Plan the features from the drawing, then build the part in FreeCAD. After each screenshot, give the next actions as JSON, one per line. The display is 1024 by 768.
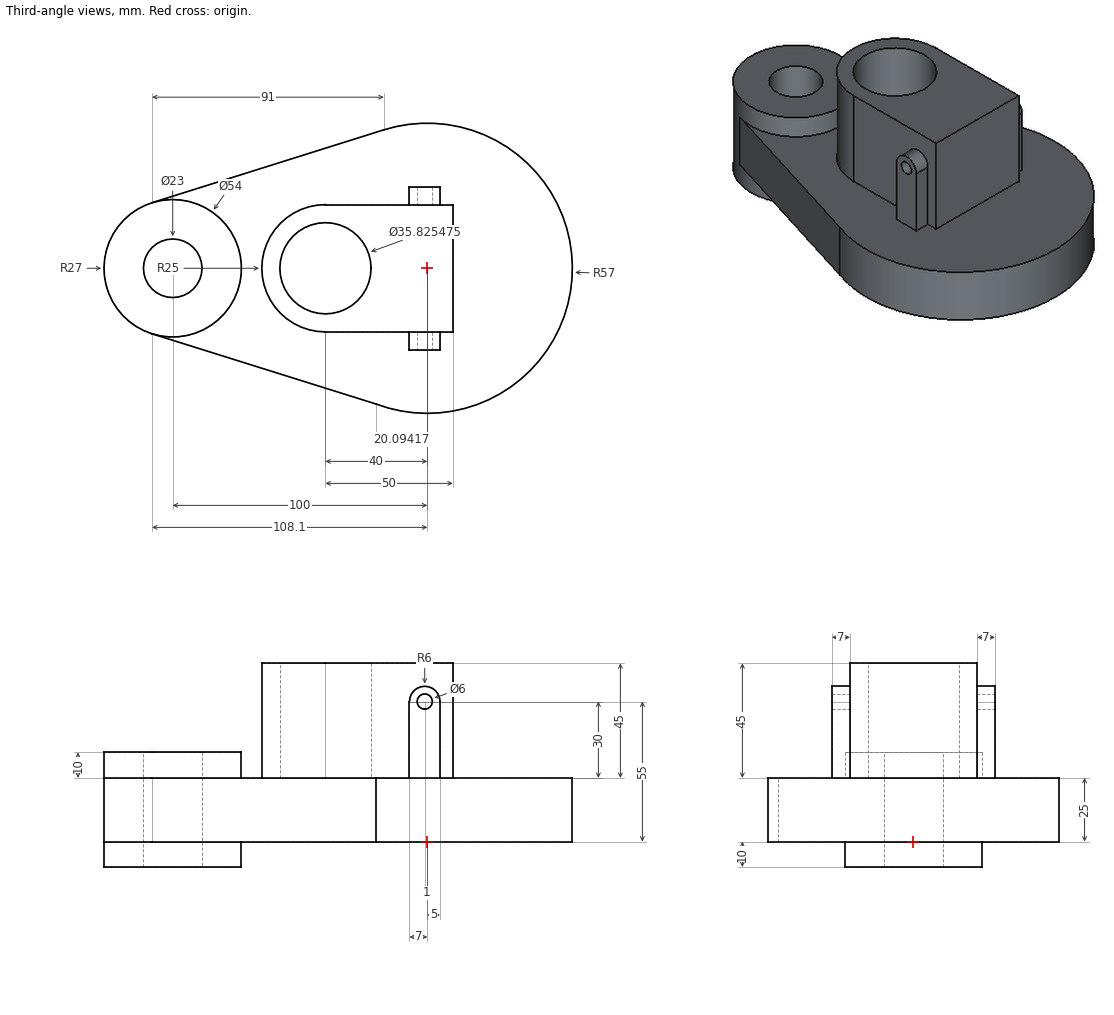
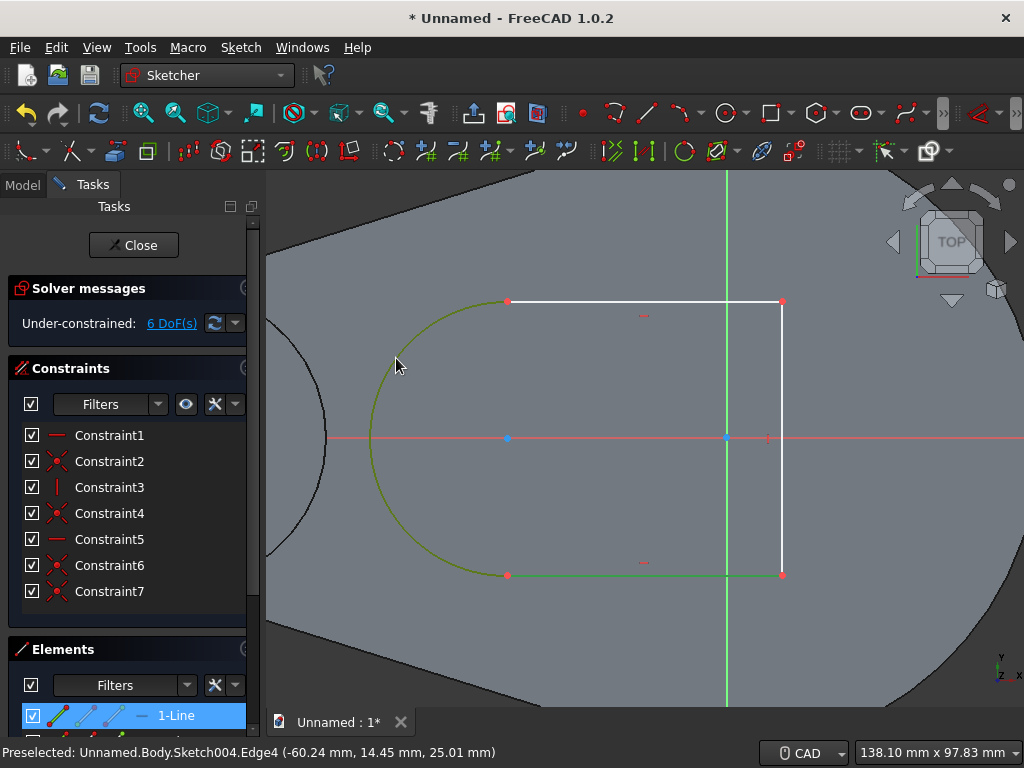
{"action": "key", "text": "t"}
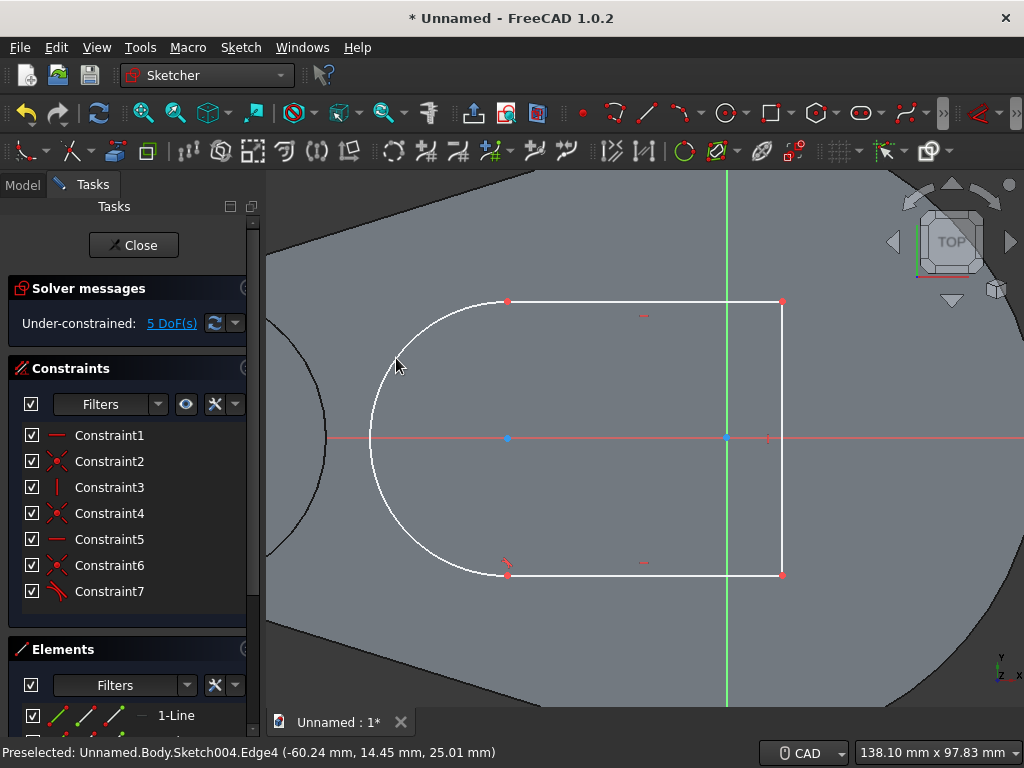
{"action": "left_click", "coordinate": [700, 302]}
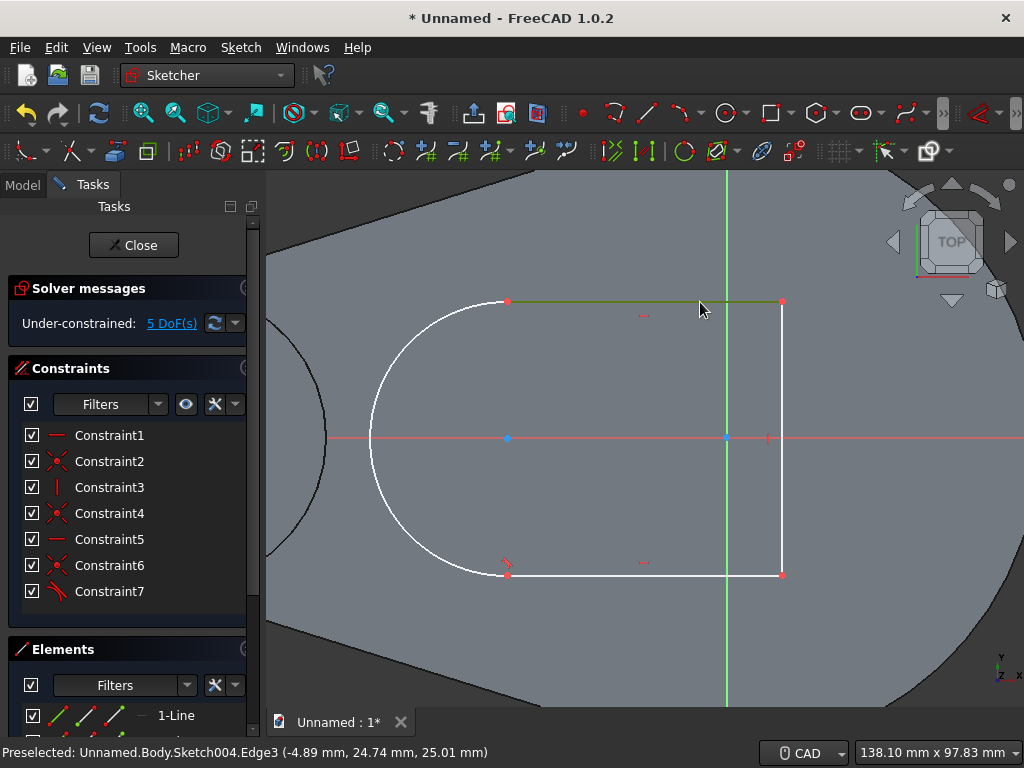
{"action": "left_click", "coordinate": [396, 359]}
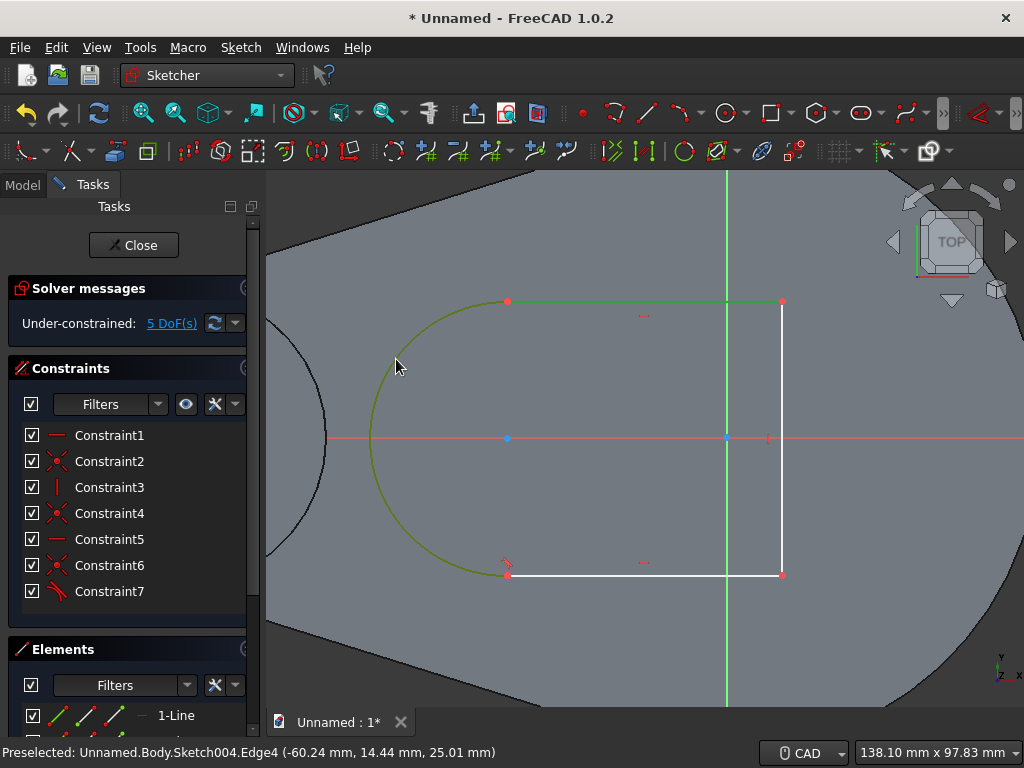
{"action": "key", "text": "t"}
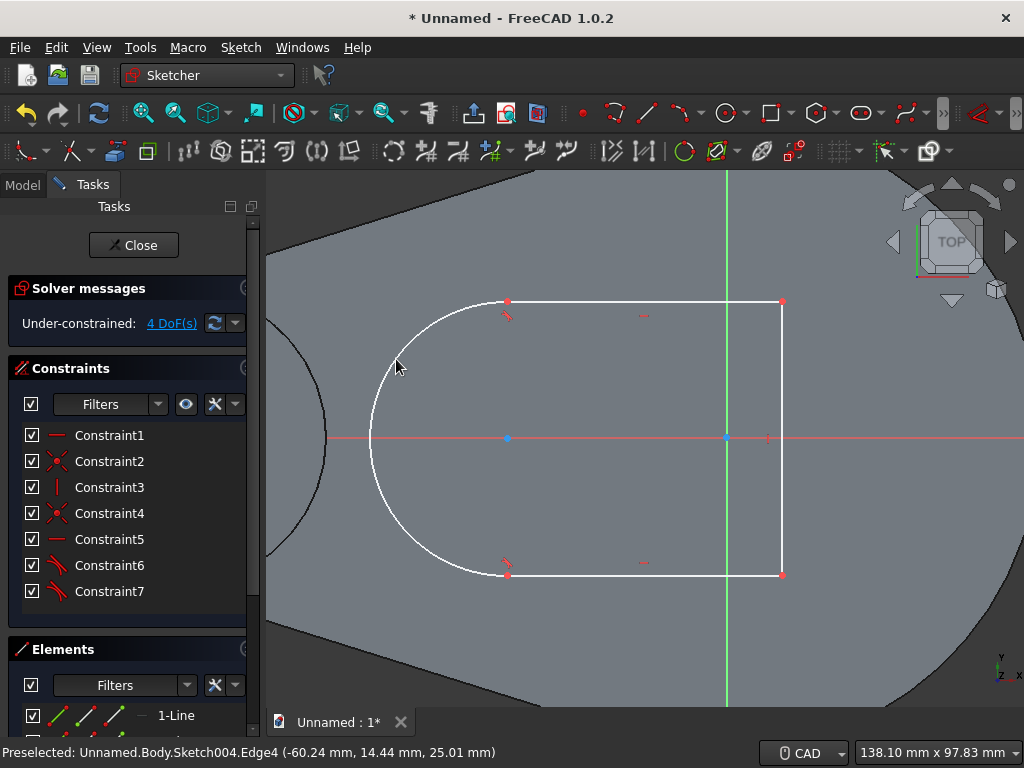
{"action": "left_click", "coordinate": [507, 439]}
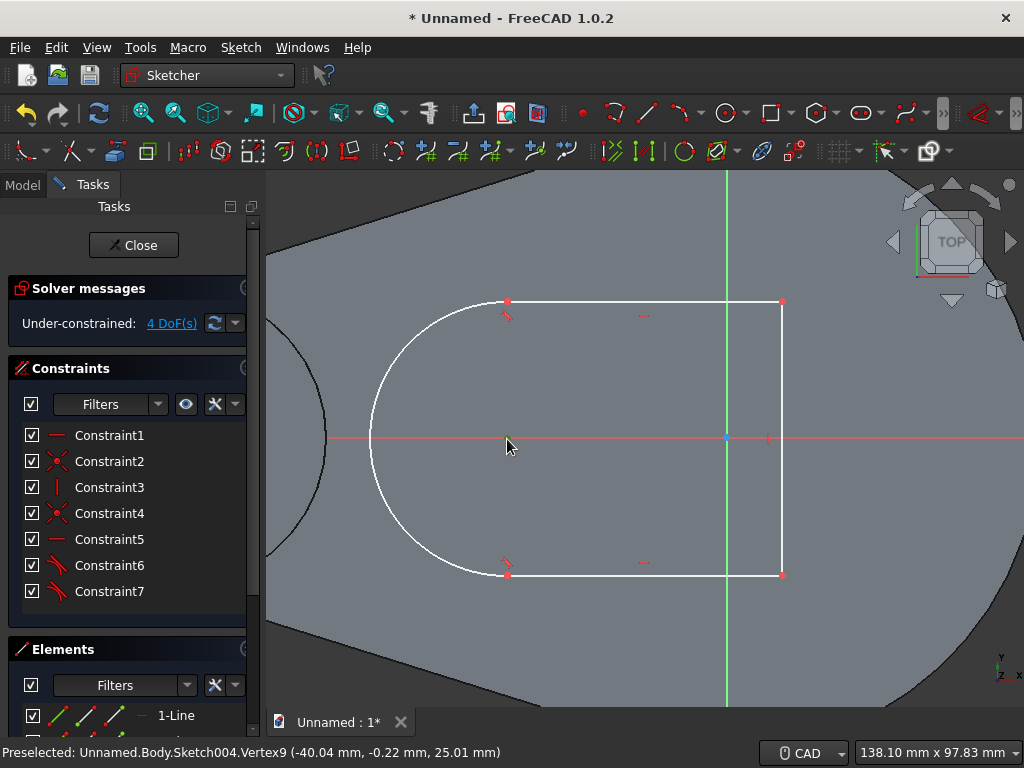
{"action": "left_click", "coordinate": [334, 438]}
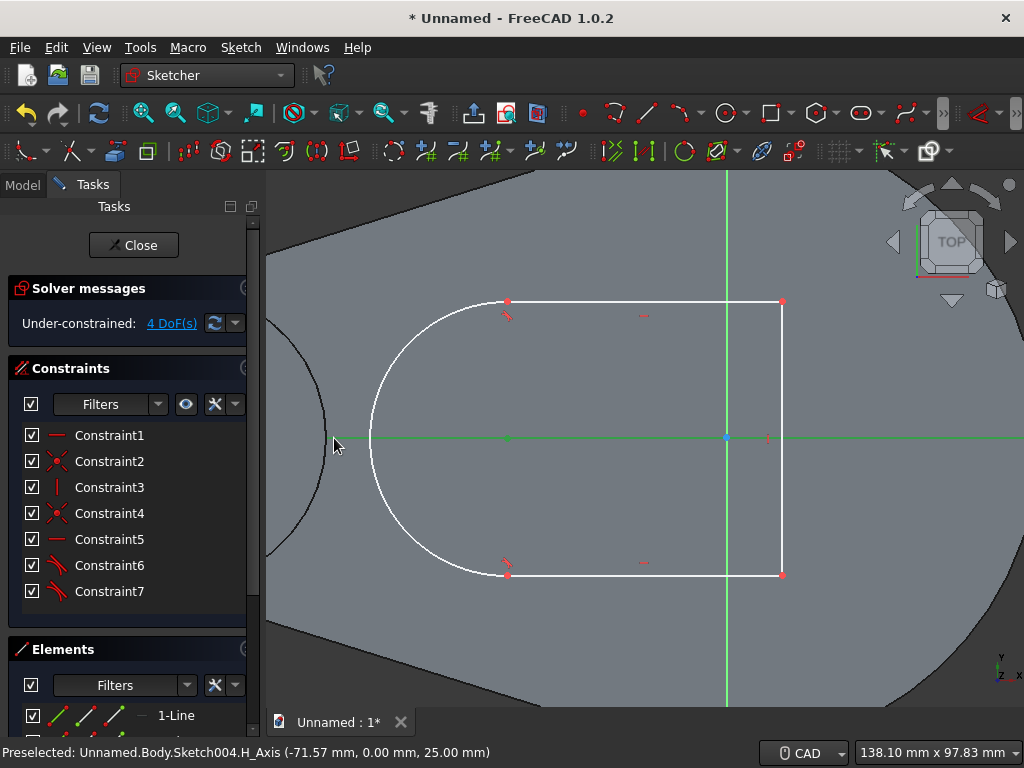
{"action": "key", "text": "c"}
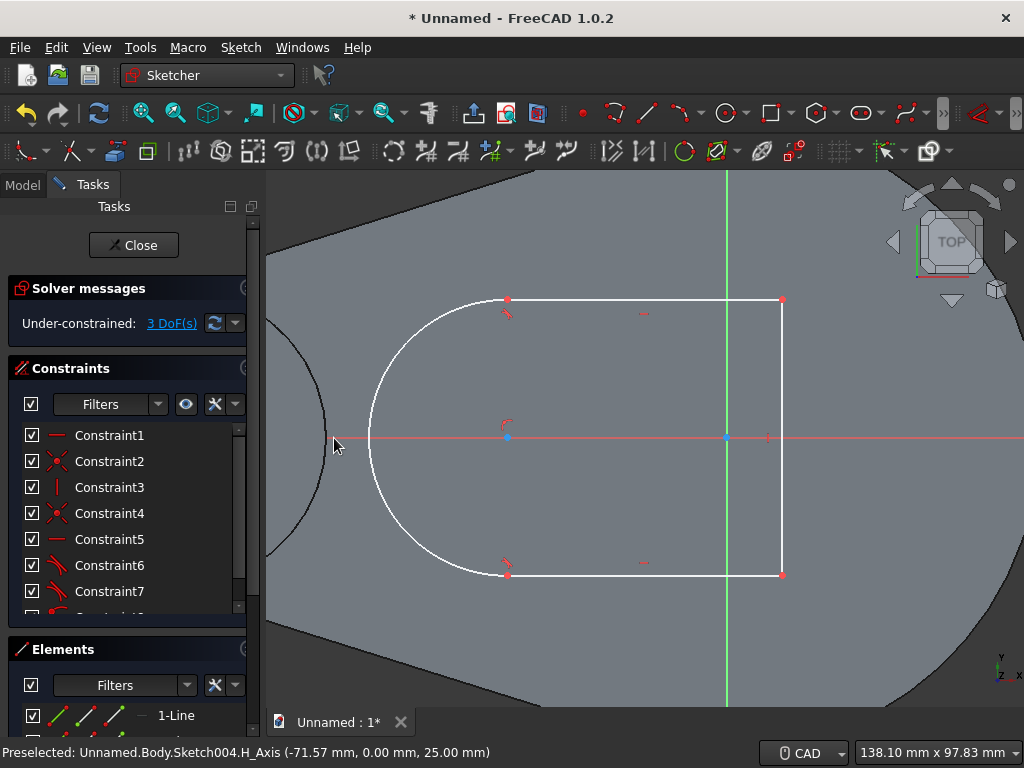
{"action": "left_click", "coordinate": [978, 114]}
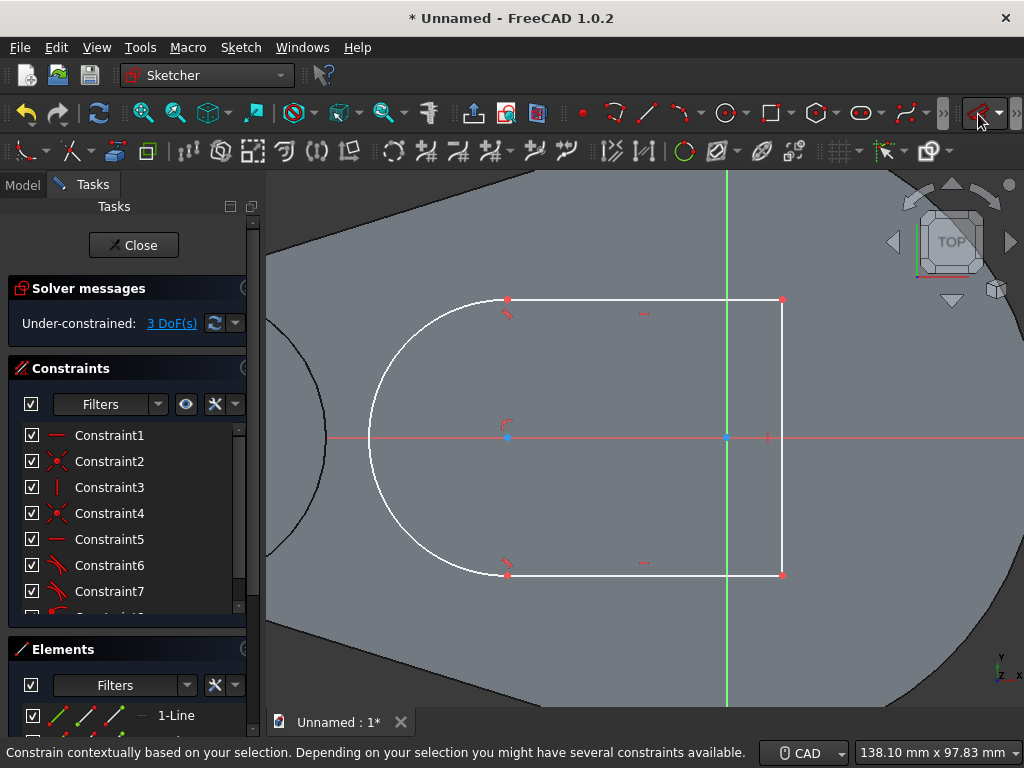
{"action": "left_click", "coordinate": [395, 357]}
{"action": "left_click", "coordinate": [369, 338]}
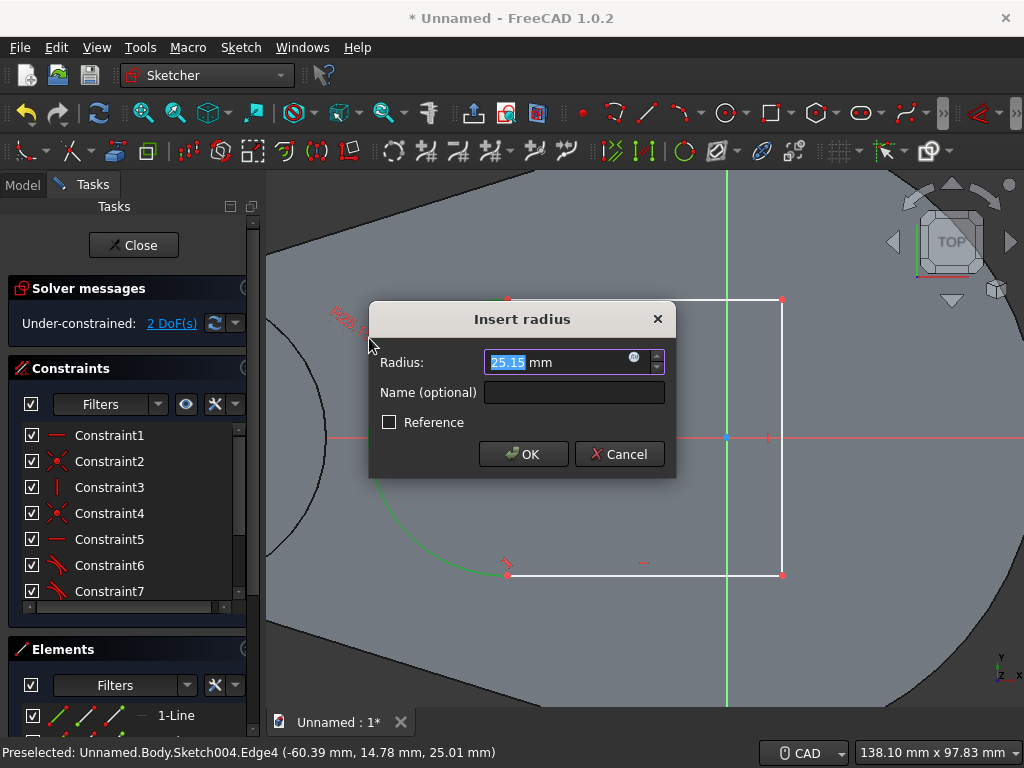
{"action": "type", "text": "25"}
{"action": "key", "text": "Return"}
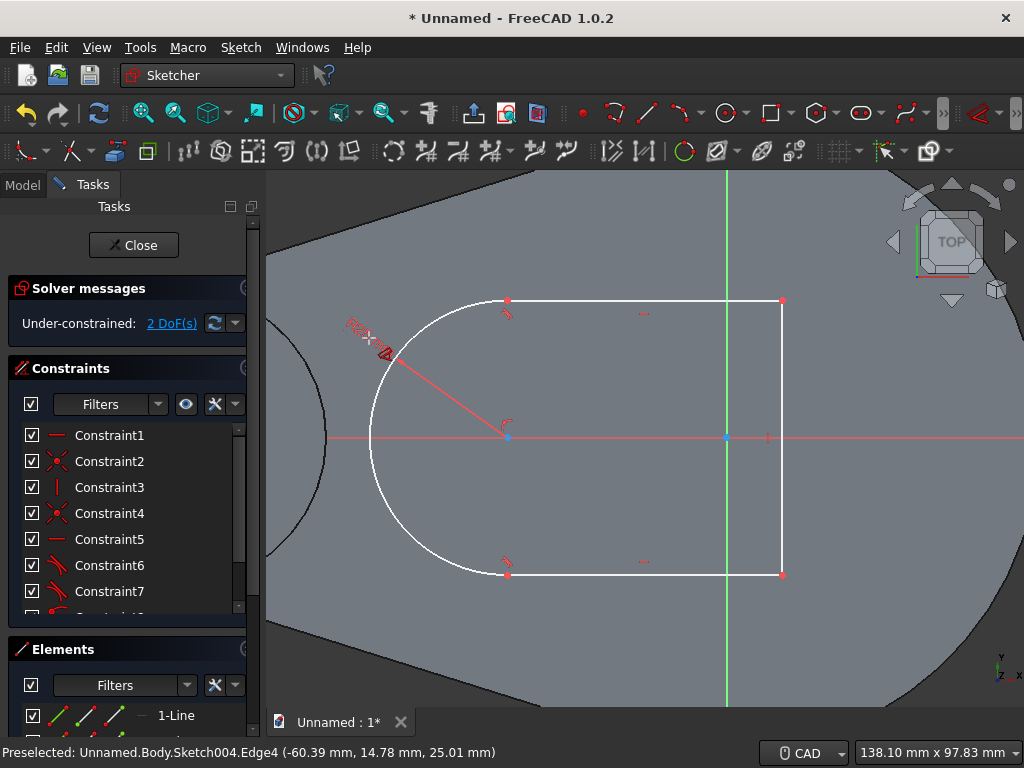
{"action": "left_click", "coordinate": [590, 575]}
{"action": "left_click", "coordinate": [645, 609]}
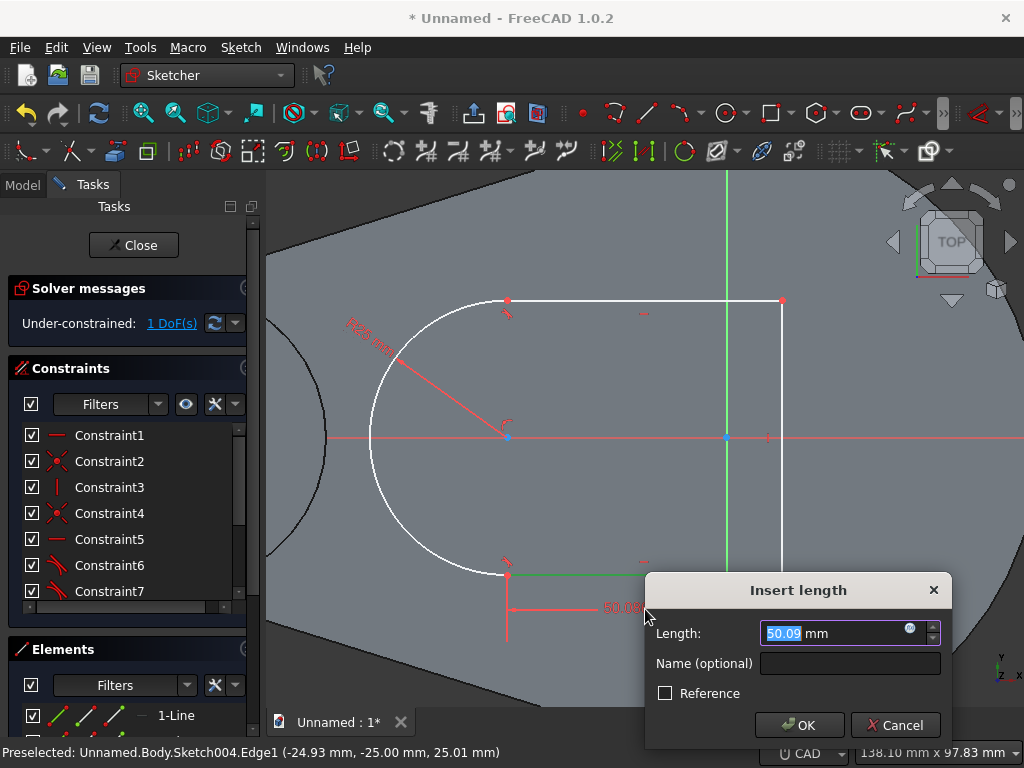
{"action": "type", "text": "50"}
{"action": "key", "text": "Return"}